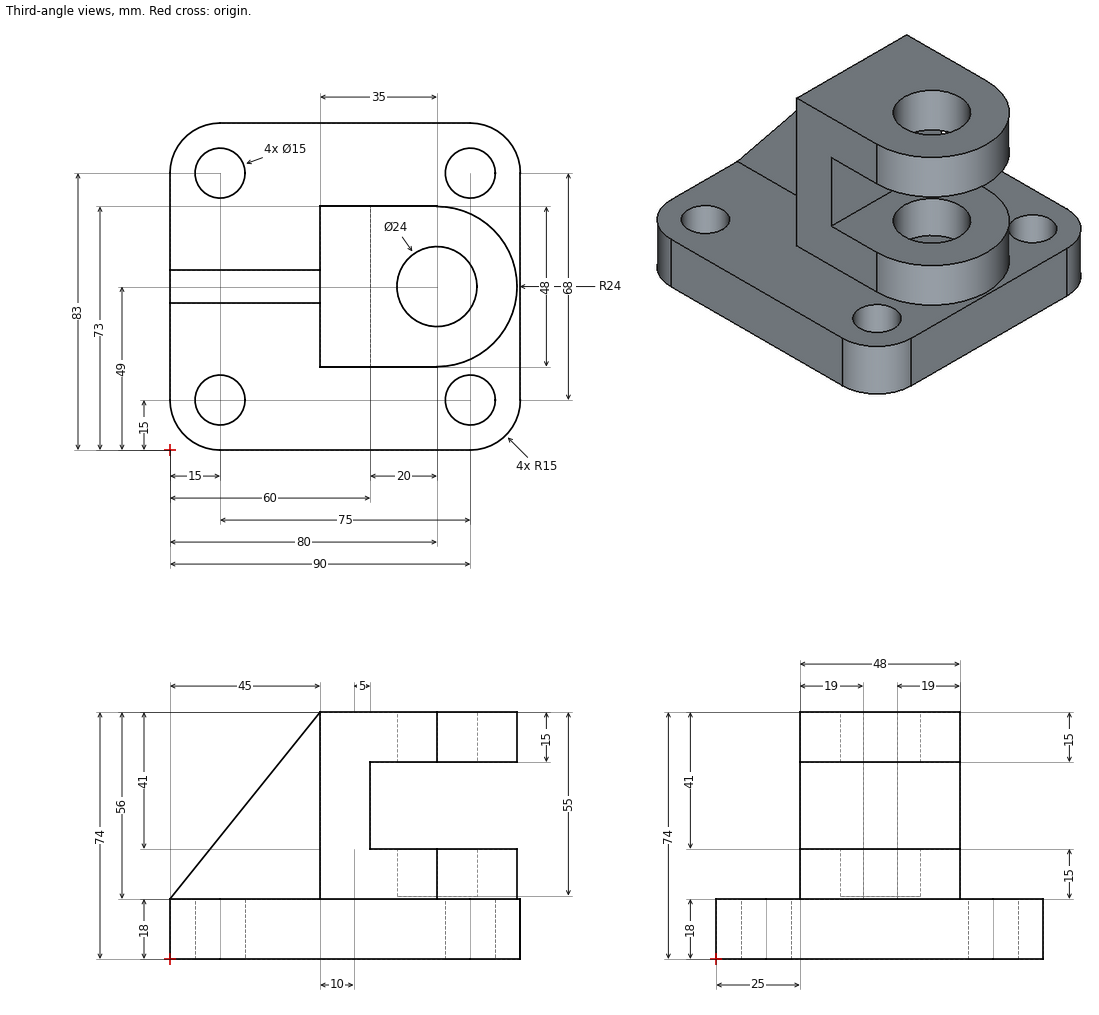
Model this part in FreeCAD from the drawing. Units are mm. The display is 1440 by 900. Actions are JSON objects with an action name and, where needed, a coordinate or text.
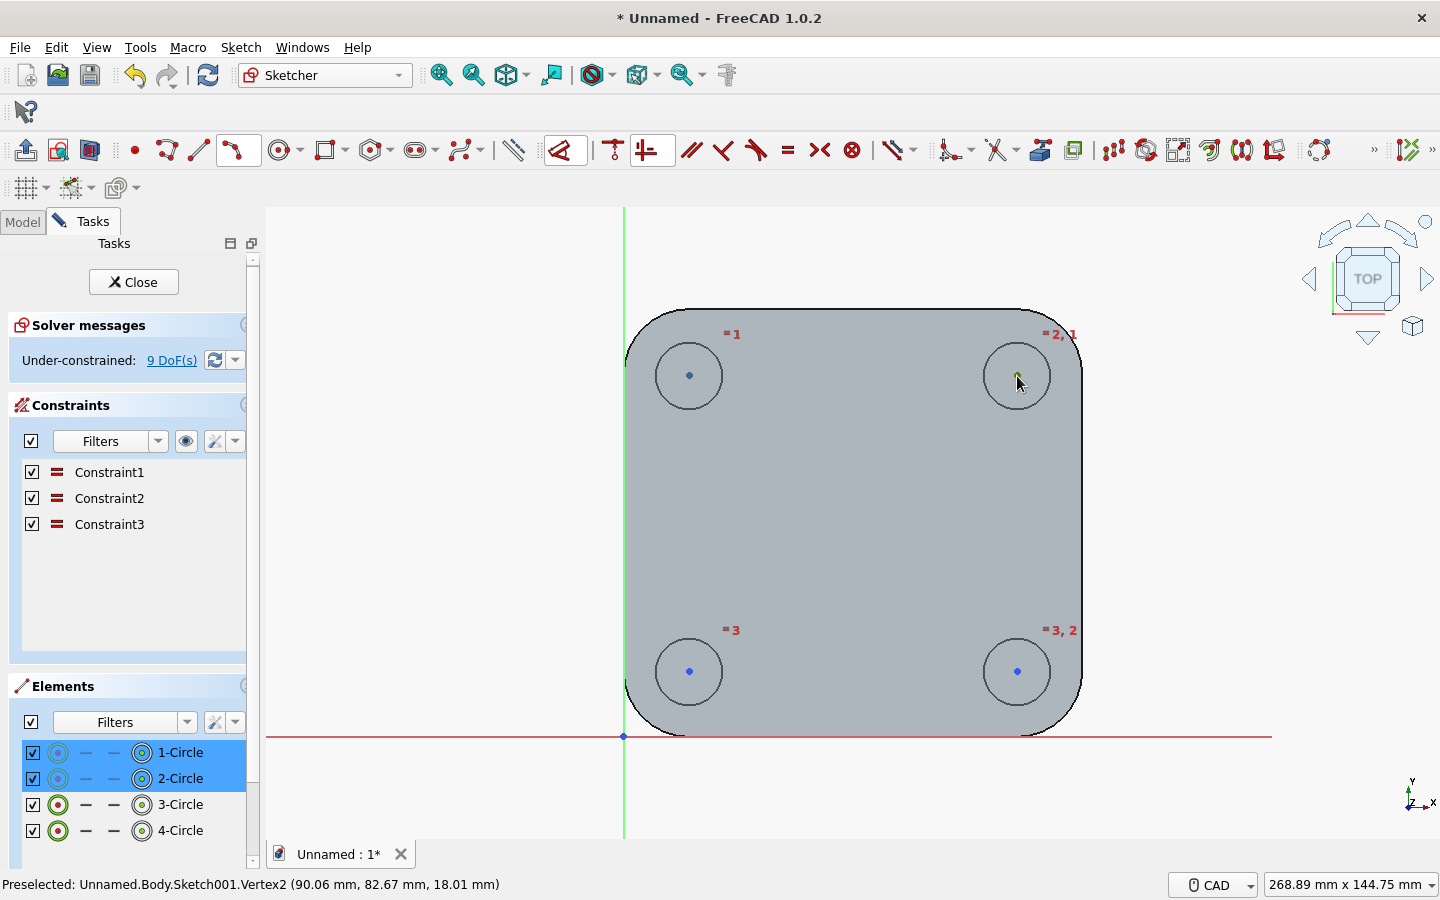
{"action": "key", "text": "h"}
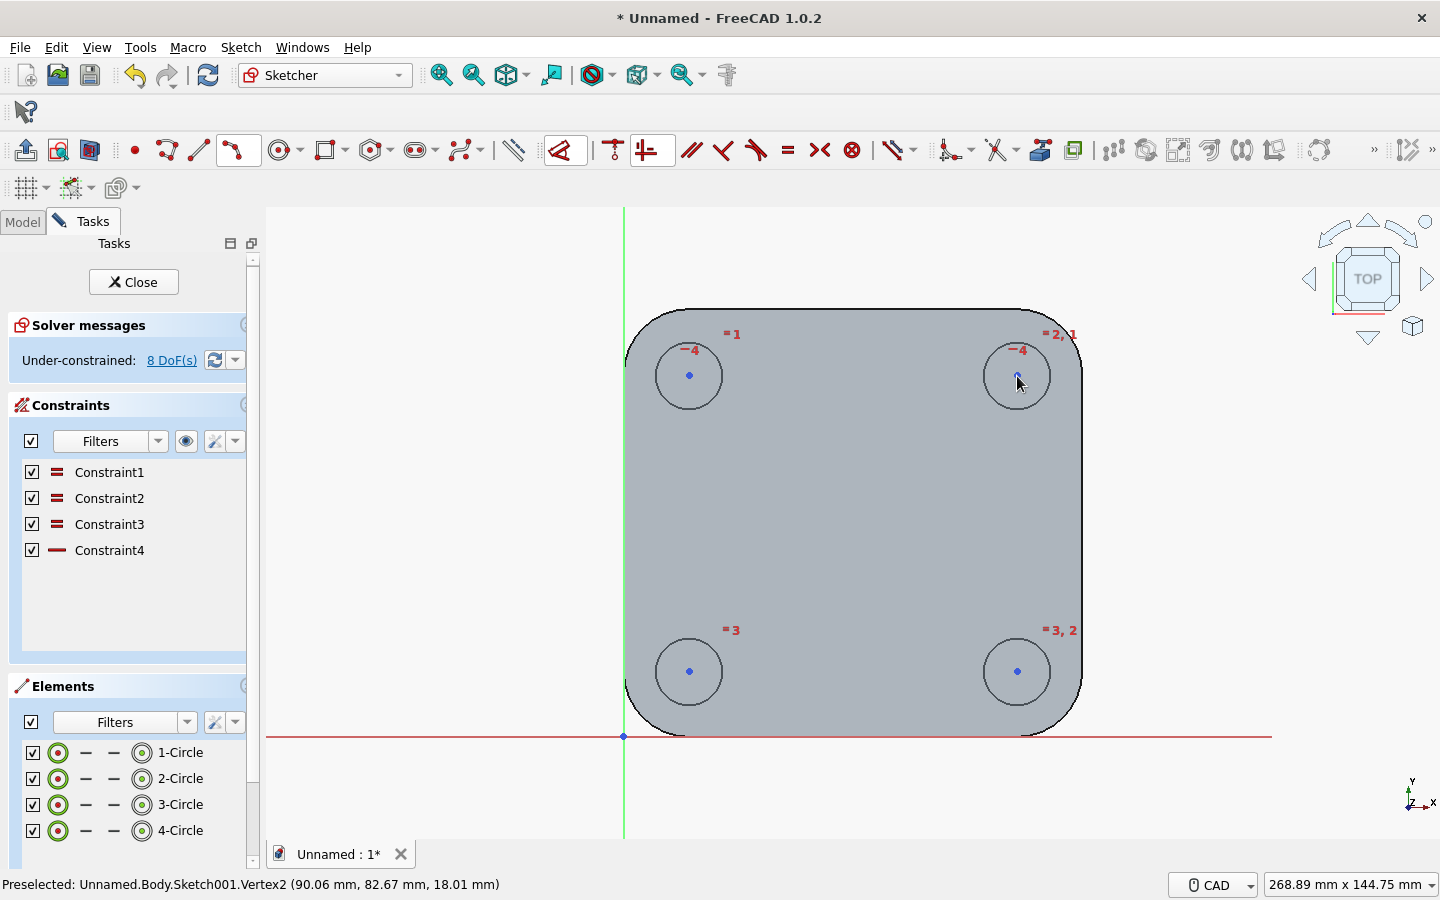
{"action": "left_click", "coordinate": [1017, 376]}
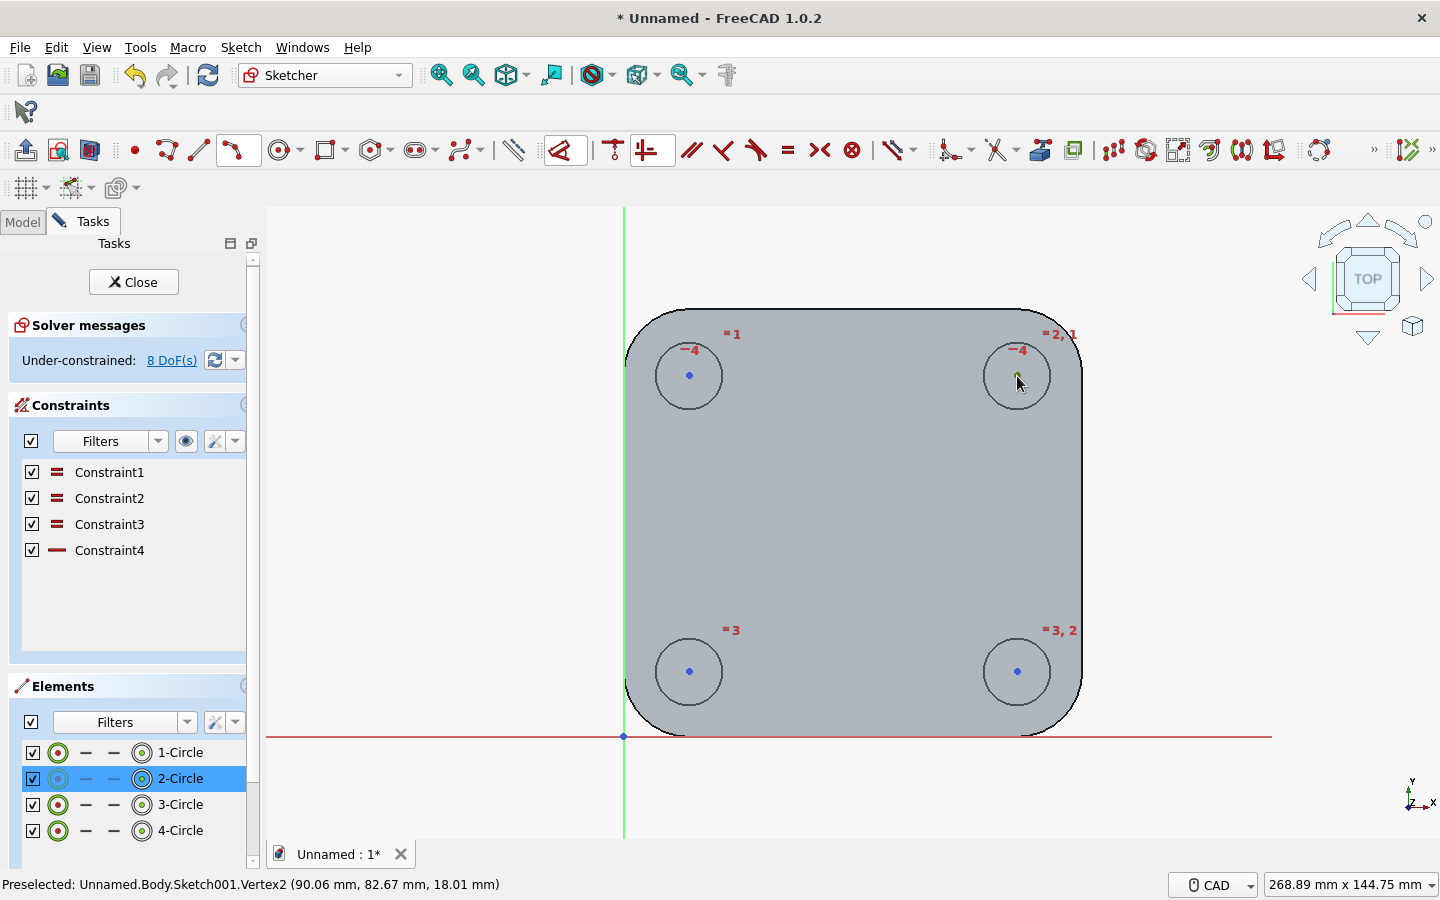
{"action": "left_click", "coordinate": [1017, 672]}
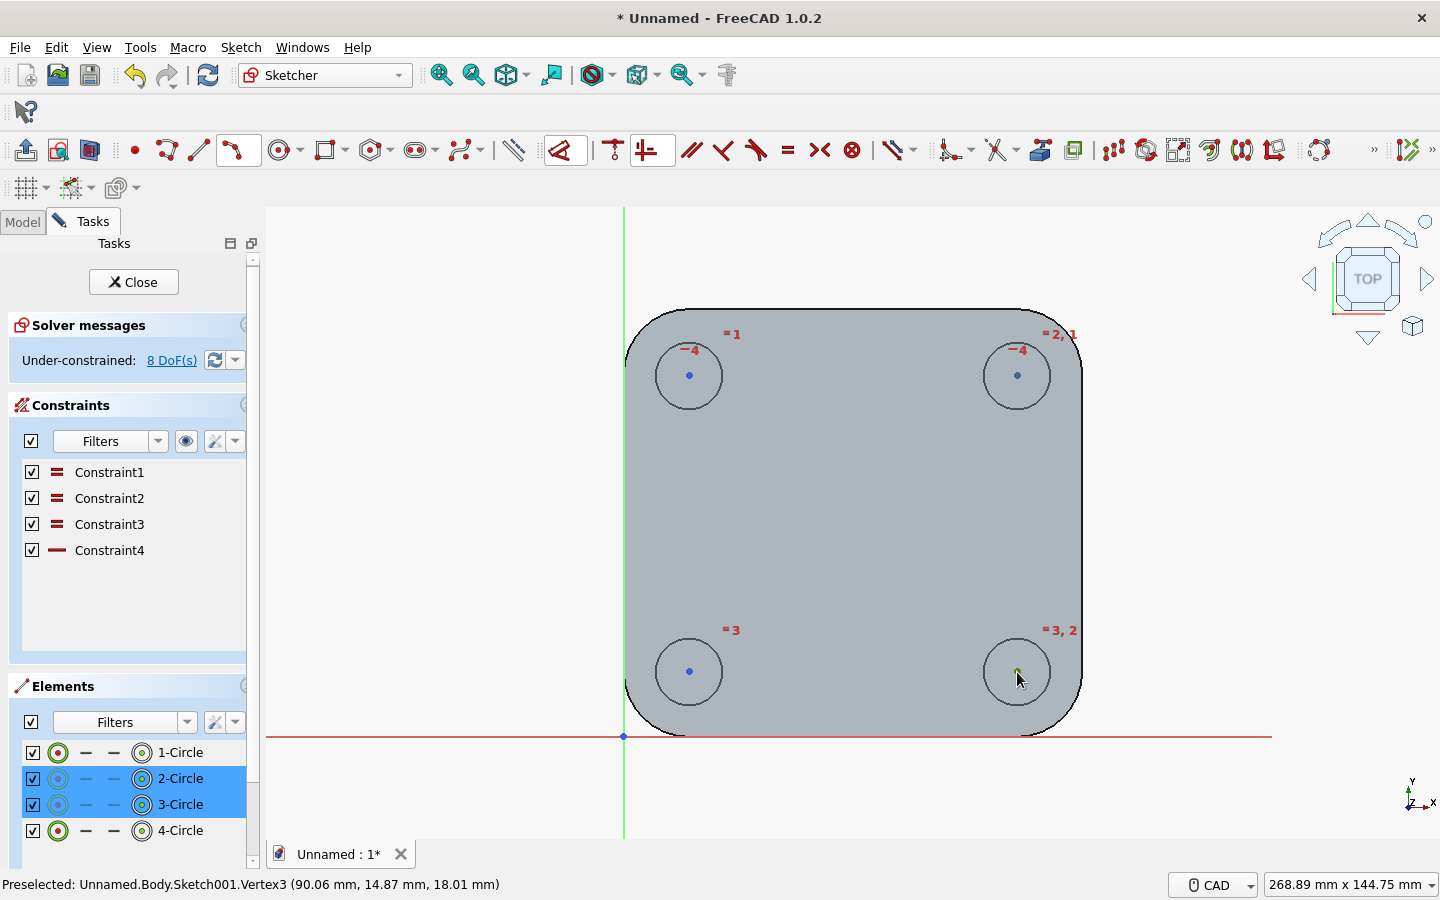
{"action": "left_click", "coordinate": [670, 150]}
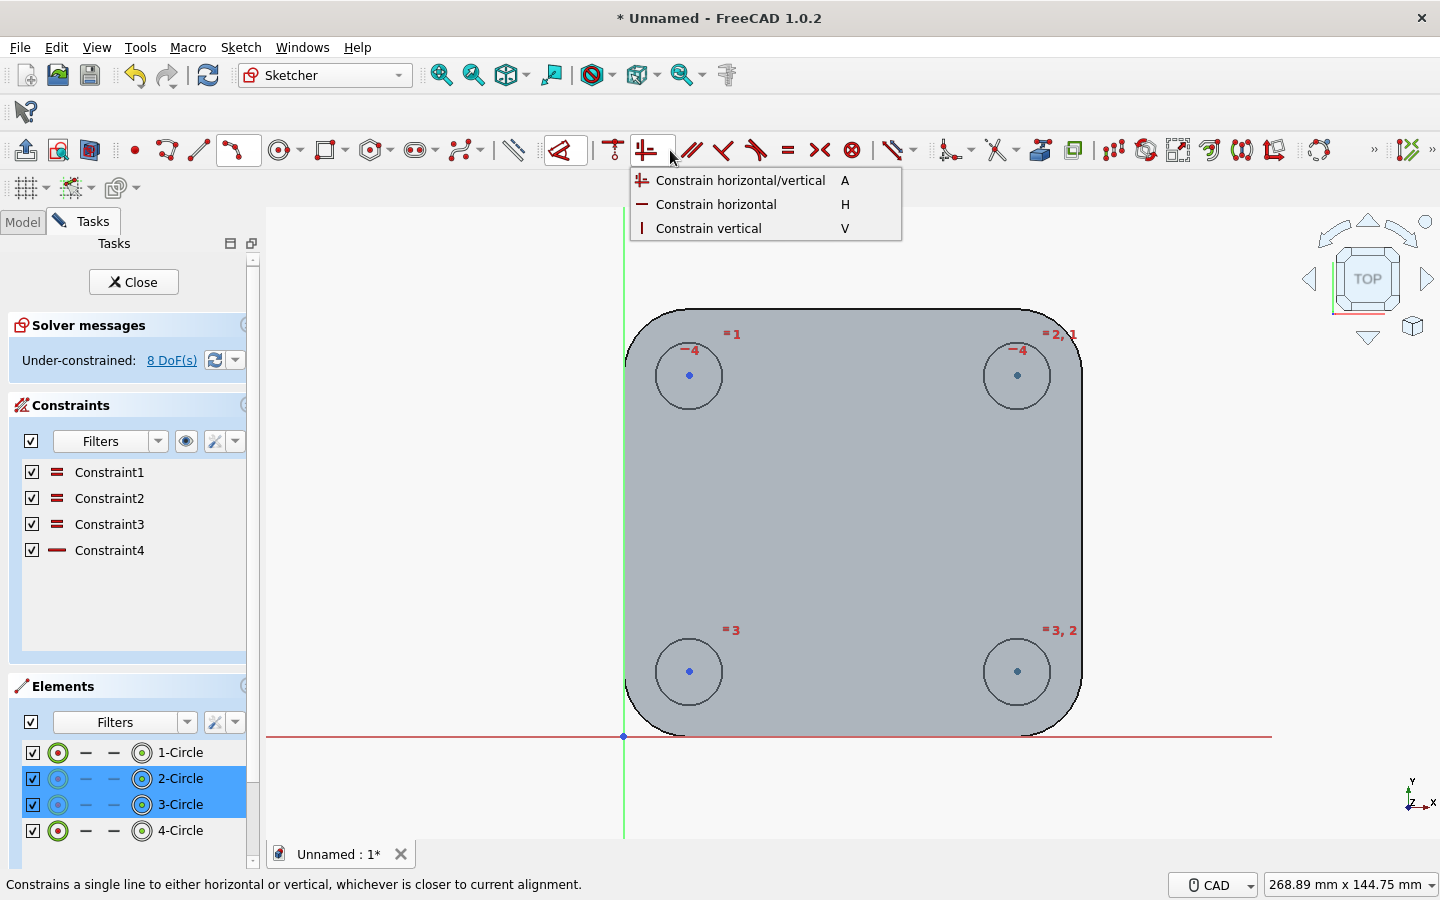
{"action": "left_click", "coordinate": [766, 228]}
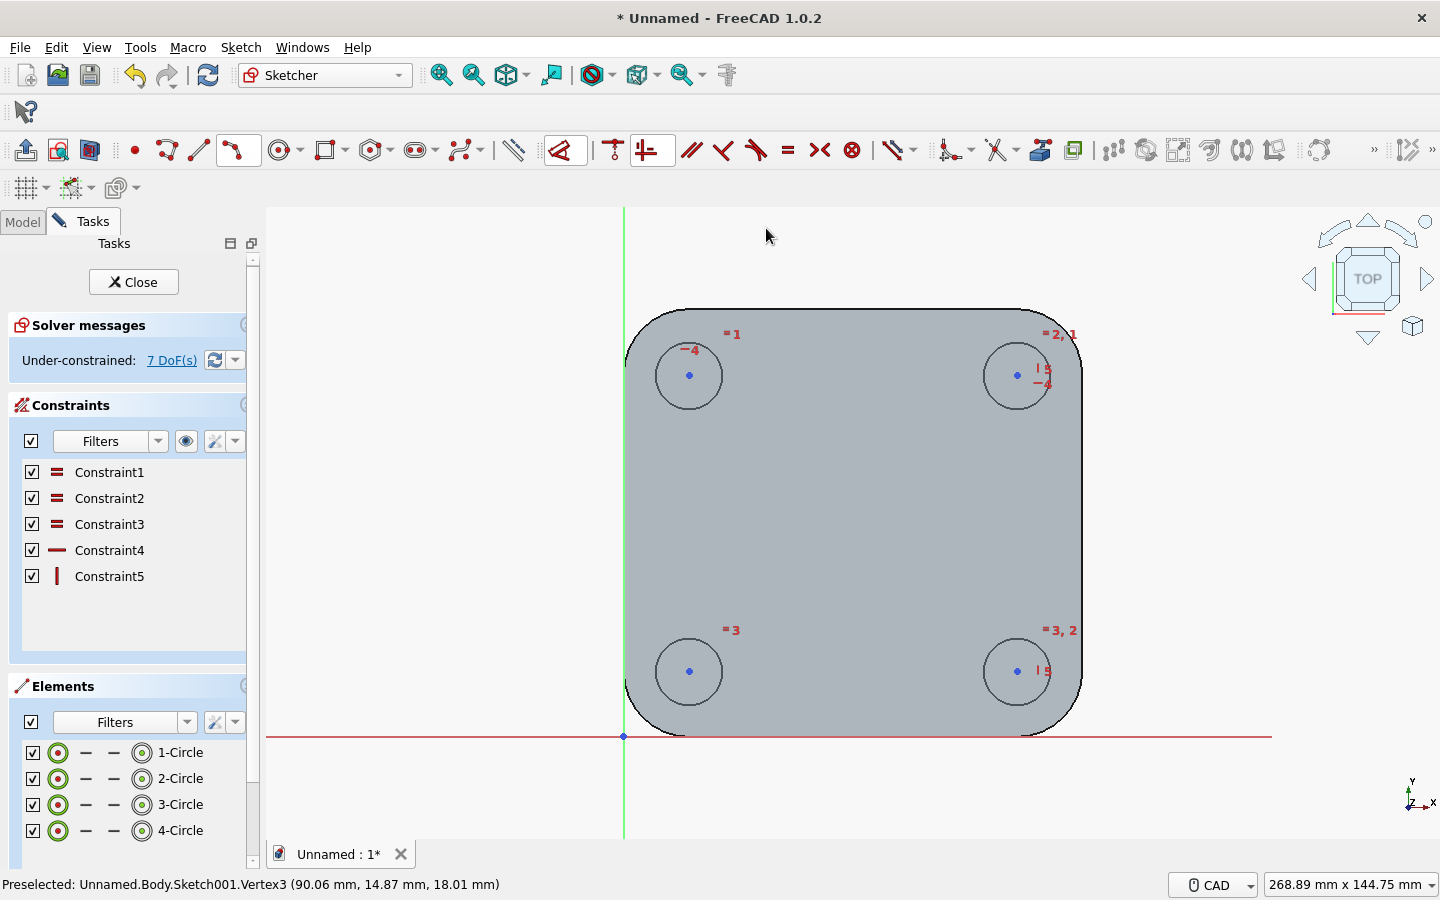
{"action": "left_click", "coordinate": [689, 376]}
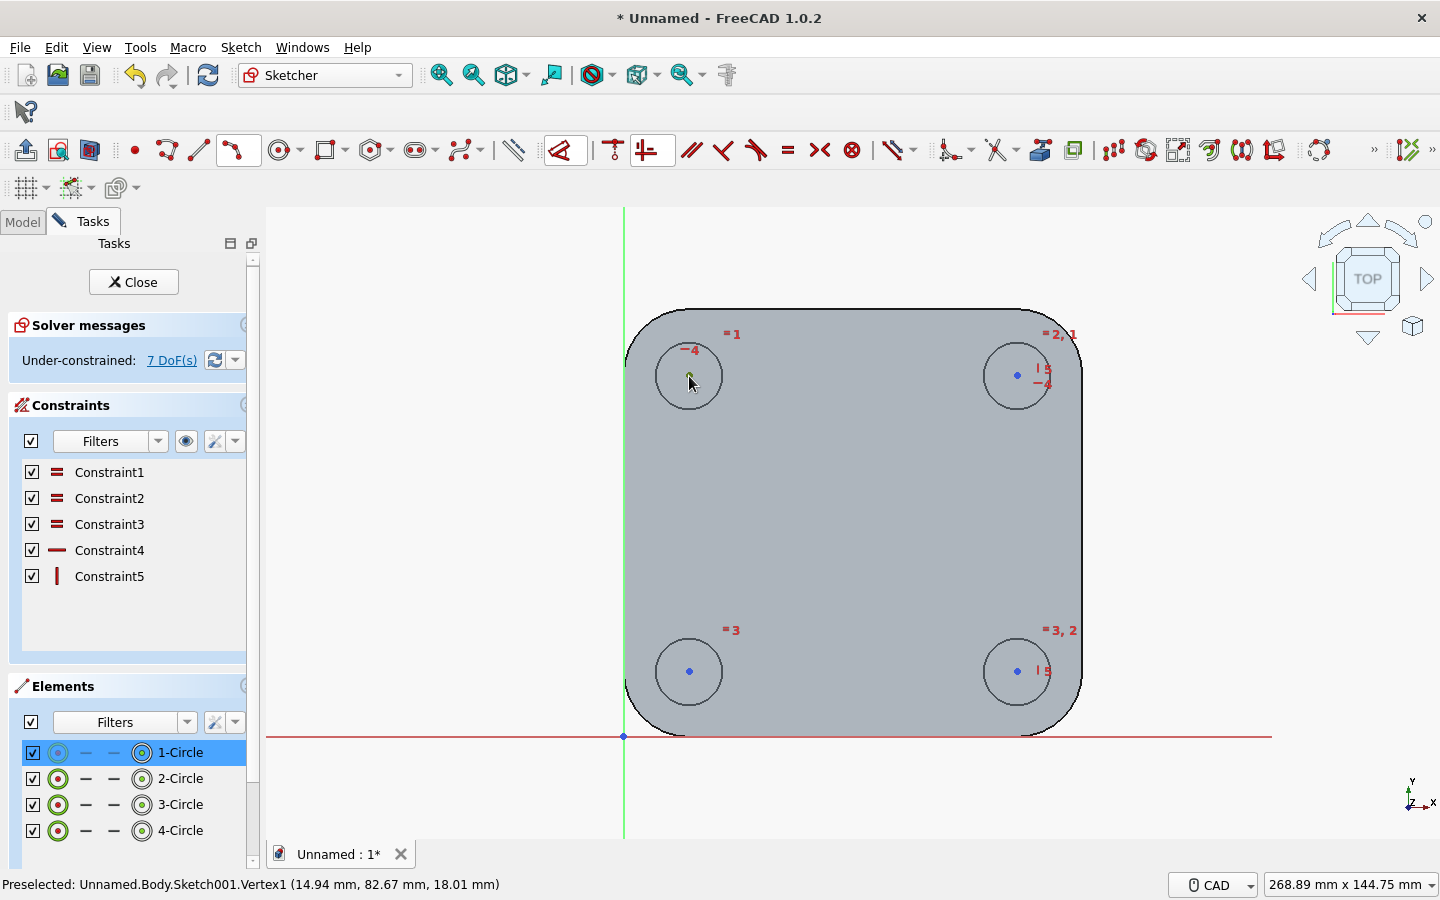
{"action": "left_click", "coordinate": [689, 672]}